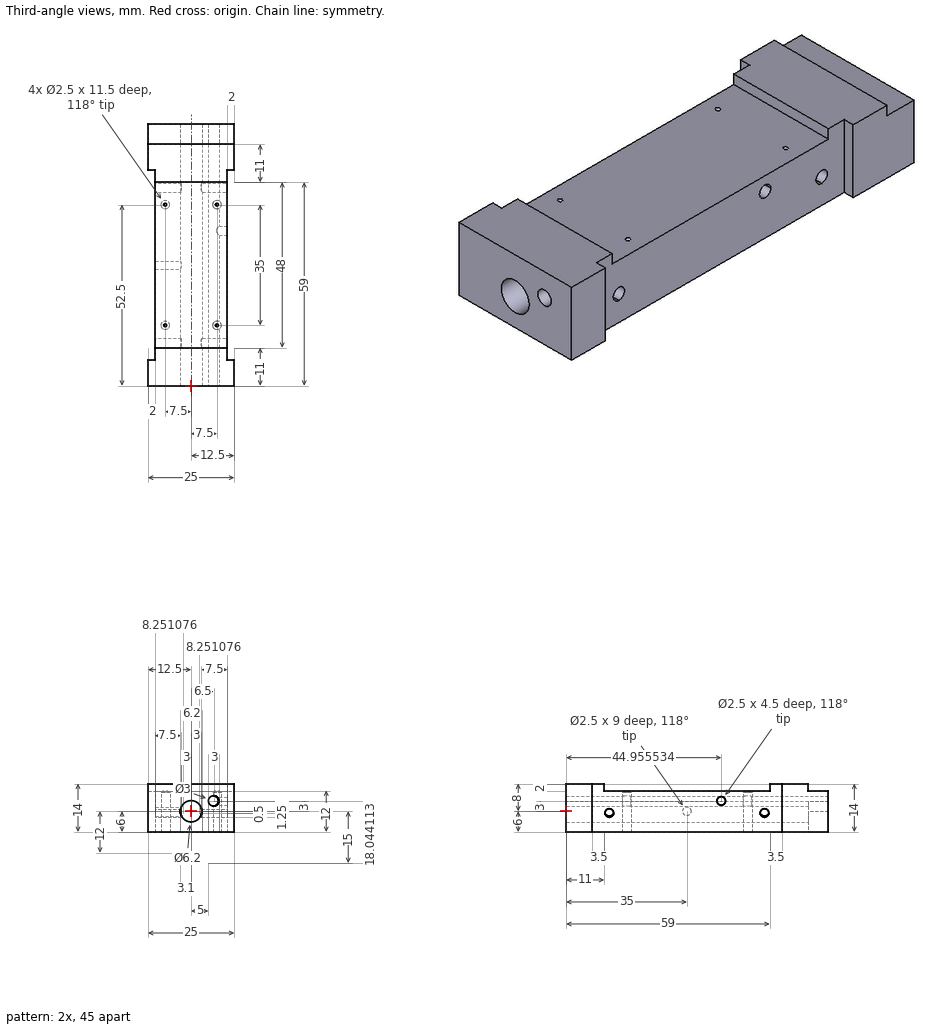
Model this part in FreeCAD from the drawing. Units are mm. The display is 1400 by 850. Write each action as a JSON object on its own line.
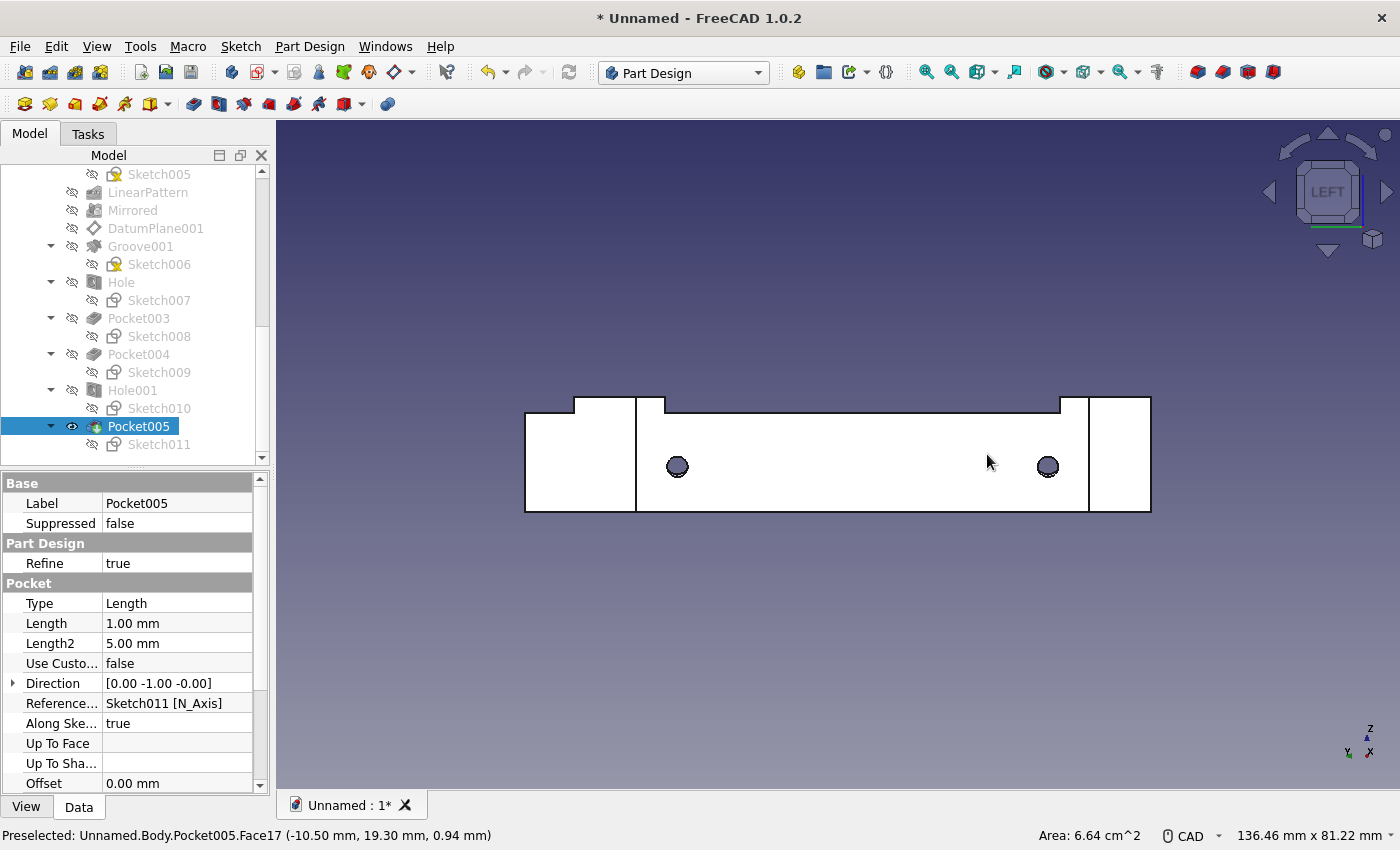
{"action": "left_click", "coordinate": [256, 72]}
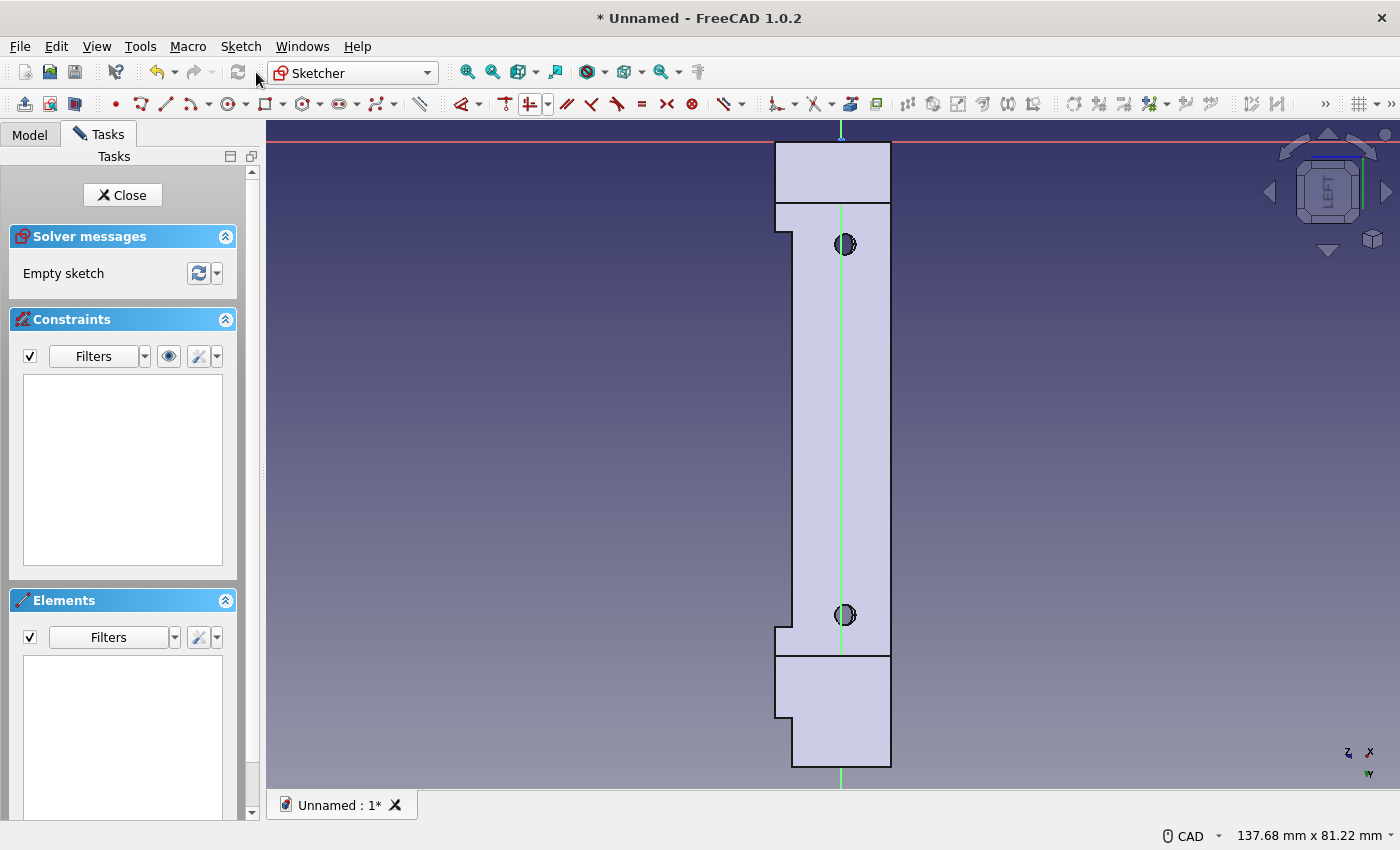
{"action": "left_click", "coordinate": [75, 104]}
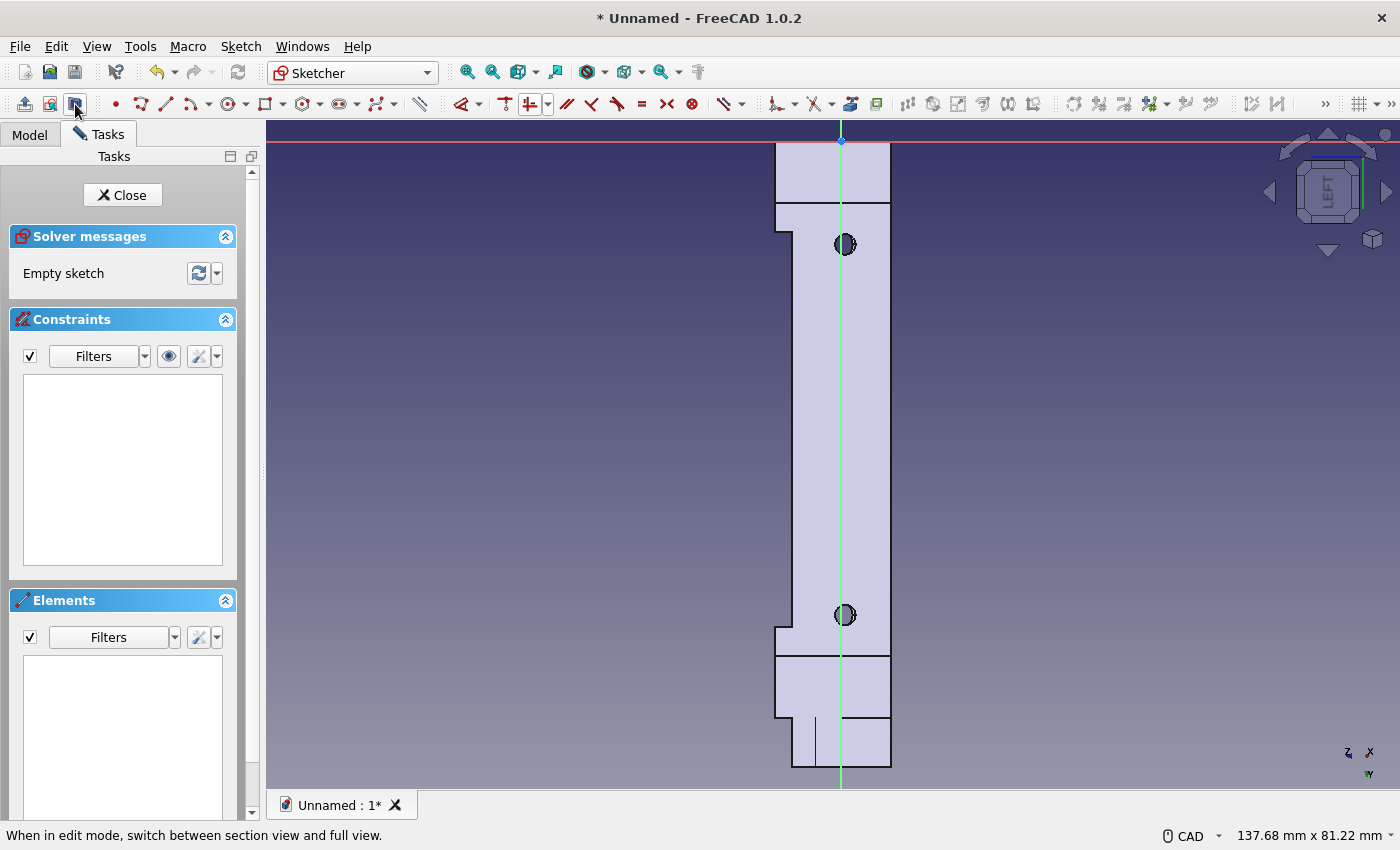
{"action": "scroll", "coordinate": [845, 428], "scroll_direction": "up", "scroll_amount": 15}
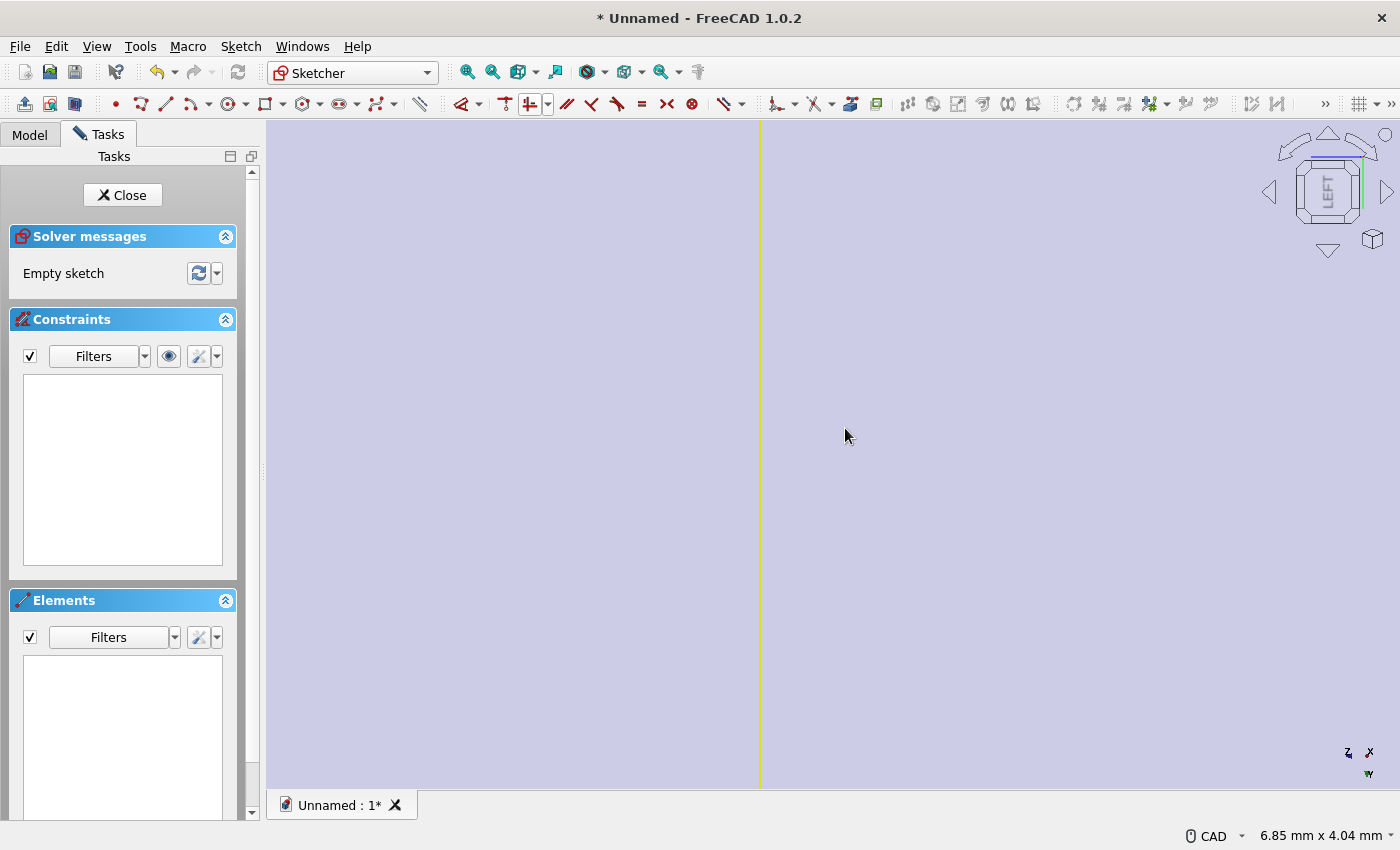
{"action": "left_click", "coordinate": [228, 104]}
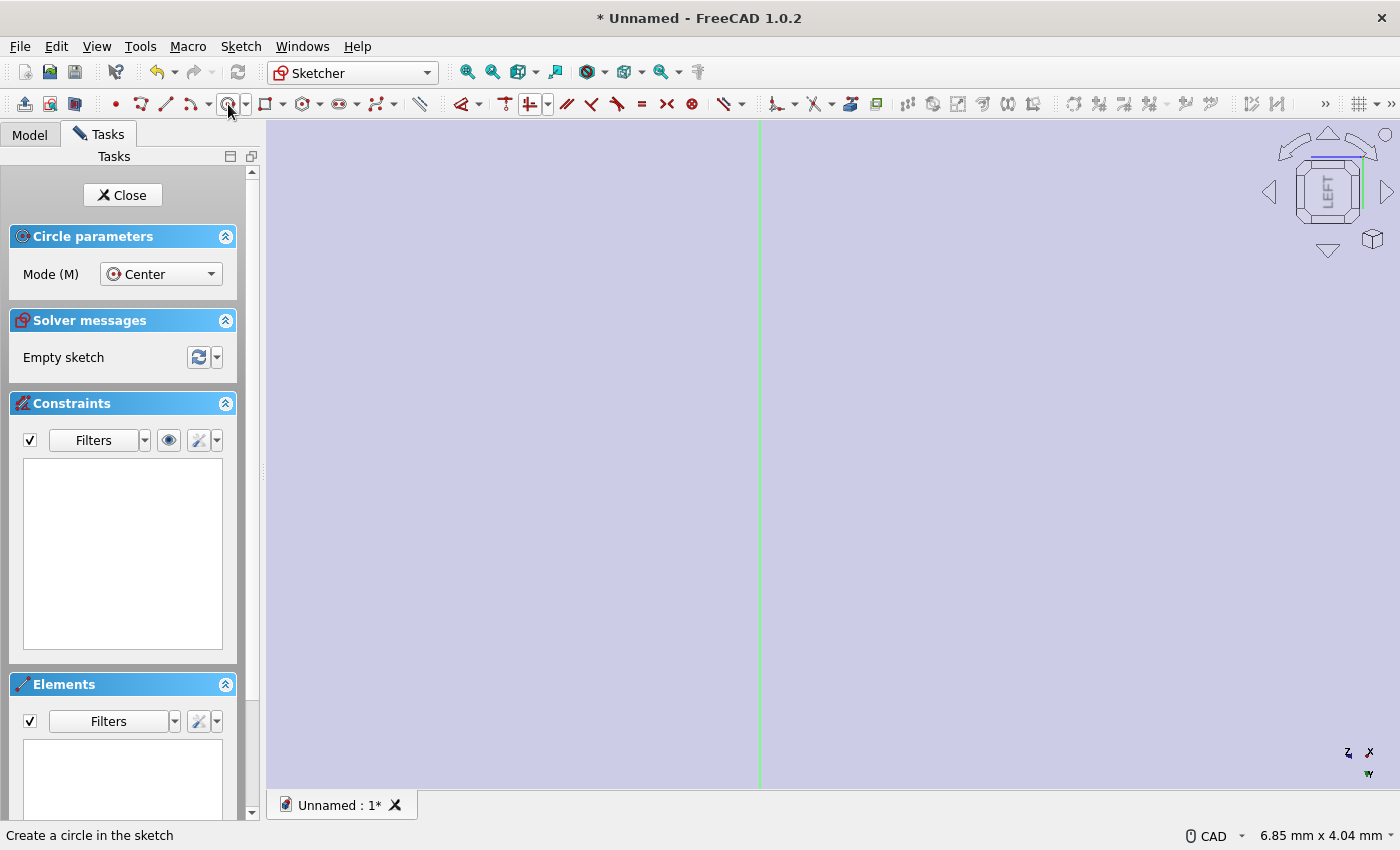
{"action": "left_click", "coordinate": [760, 455]}
{"action": "left_click", "coordinate": [906, 309]}
{"action": "key", "text": "Escape"}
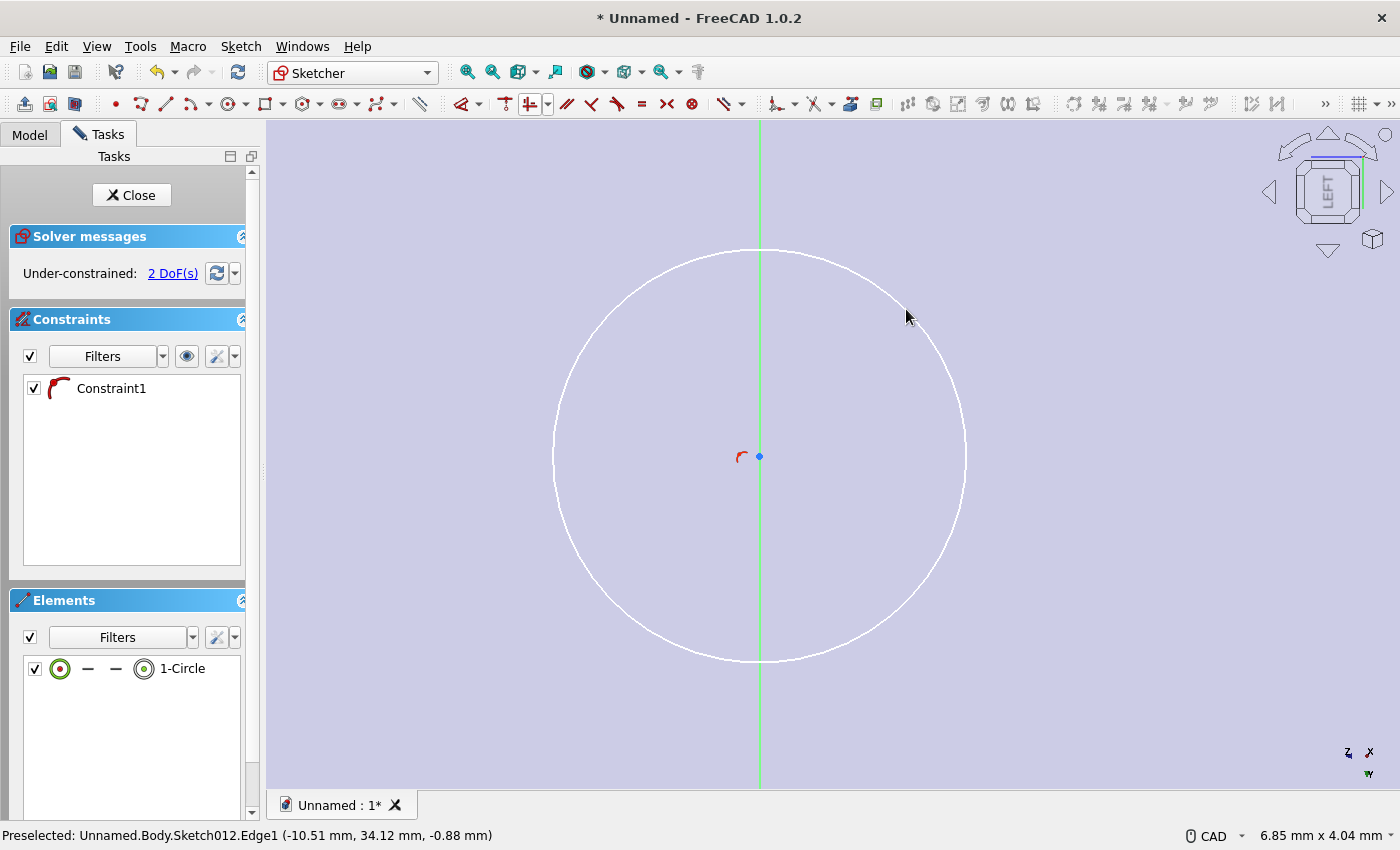
{"action": "left_click", "coordinate": [460, 104]}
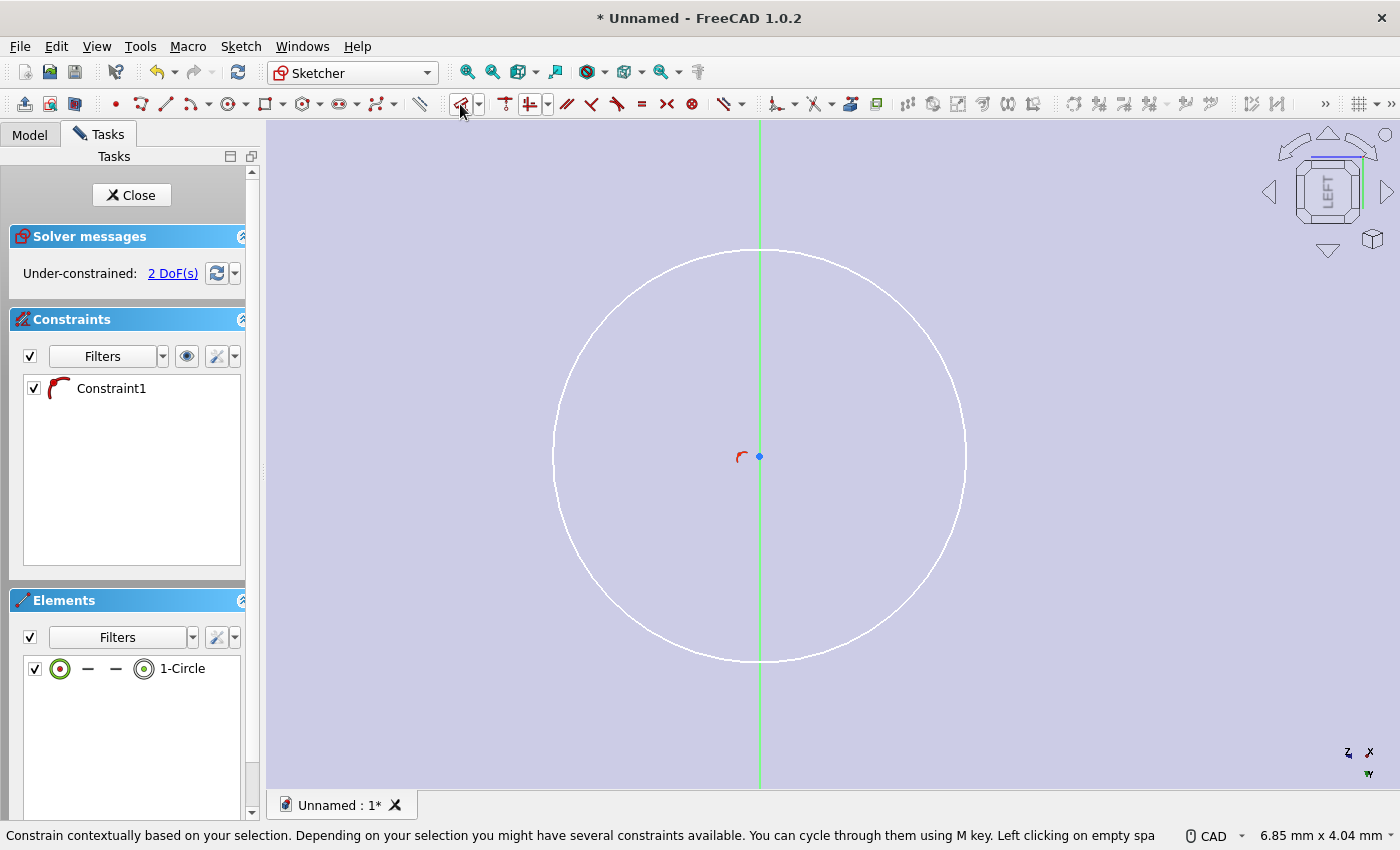
{"action": "left_click", "coordinate": [905, 309]}
{"action": "left_click", "coordinate": [927, 286]}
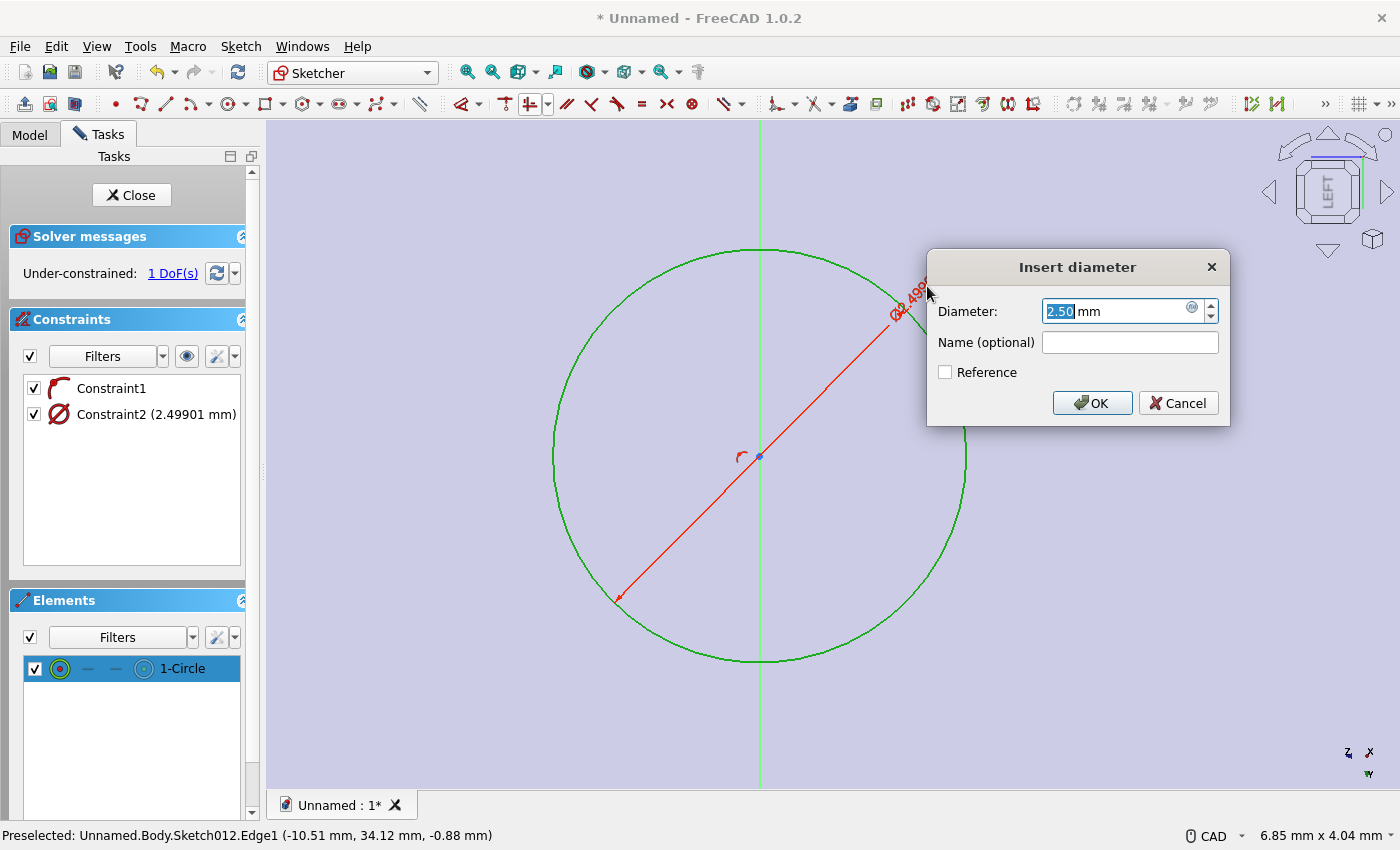
{"action": "type", "text": "2.5"}
{"action": "key", "text": "Return"}